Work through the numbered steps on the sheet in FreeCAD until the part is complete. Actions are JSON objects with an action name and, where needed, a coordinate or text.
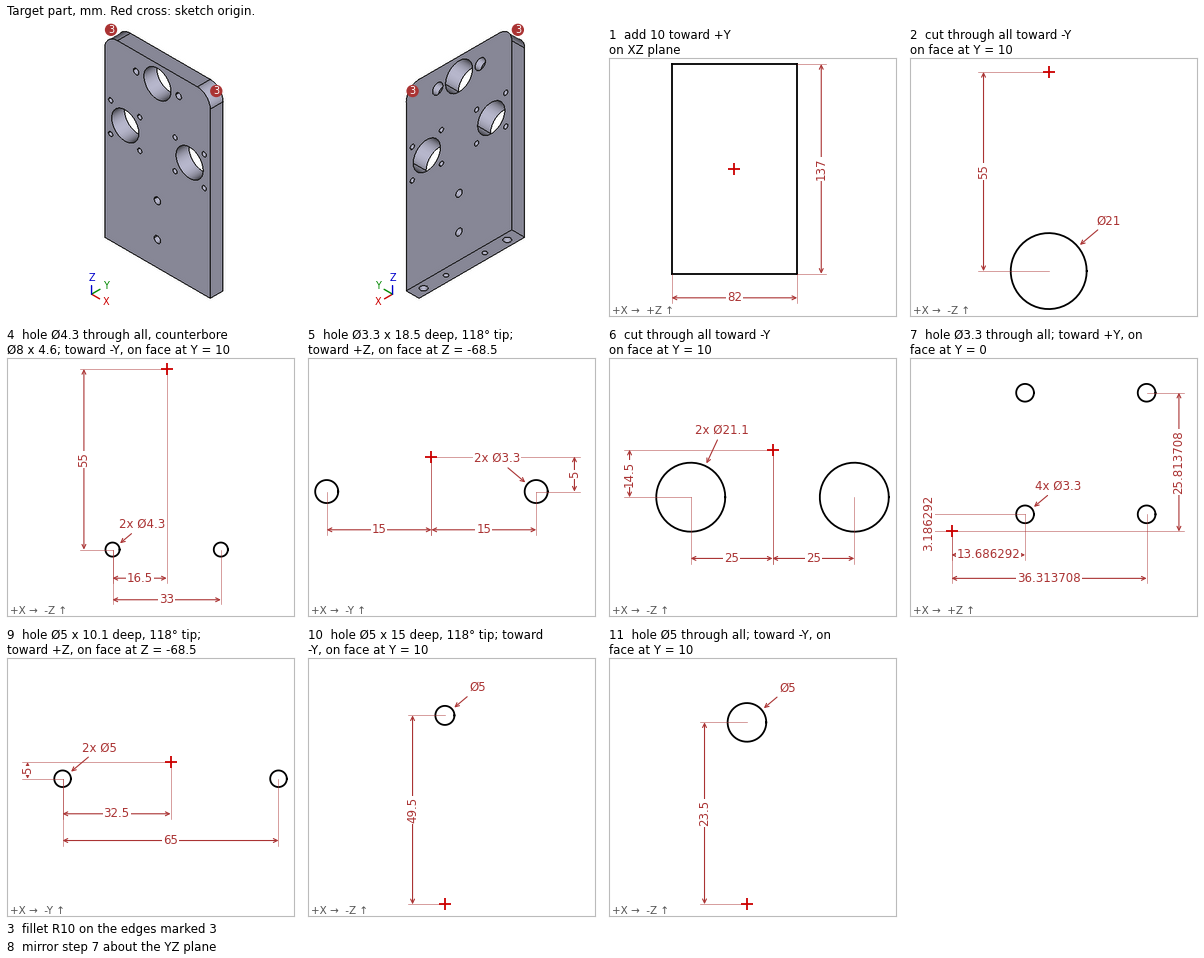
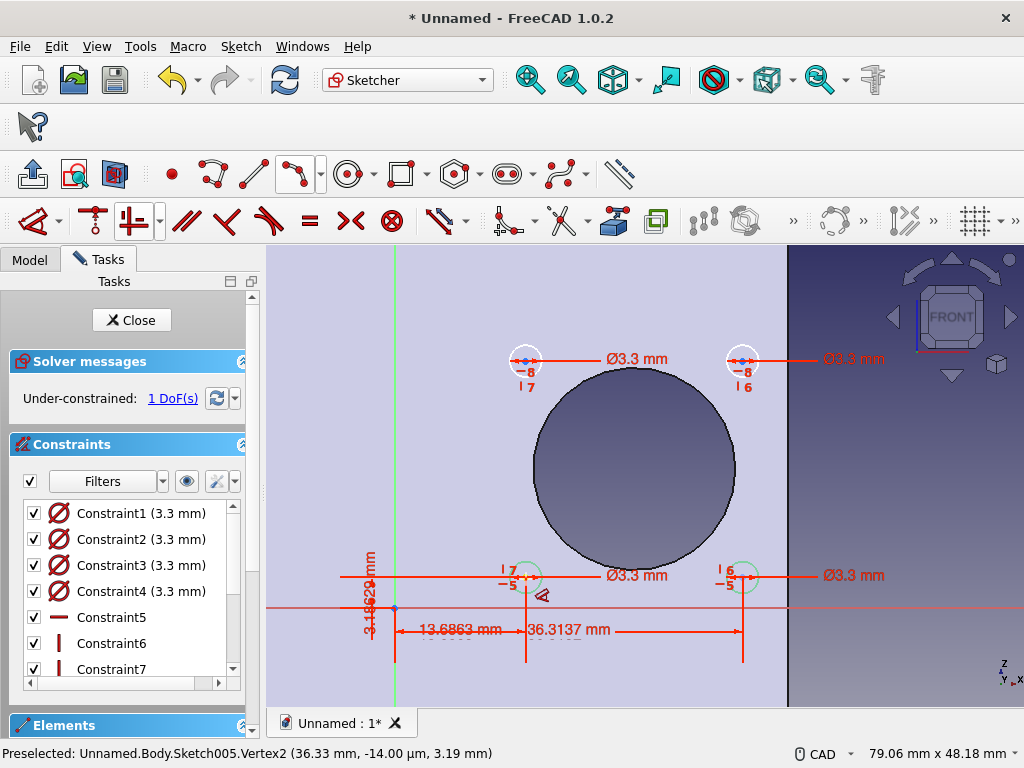
{"action": "left_click", "coordinate": [743, 361]}
{"action": "left_click", "coordinate": [361, 485]}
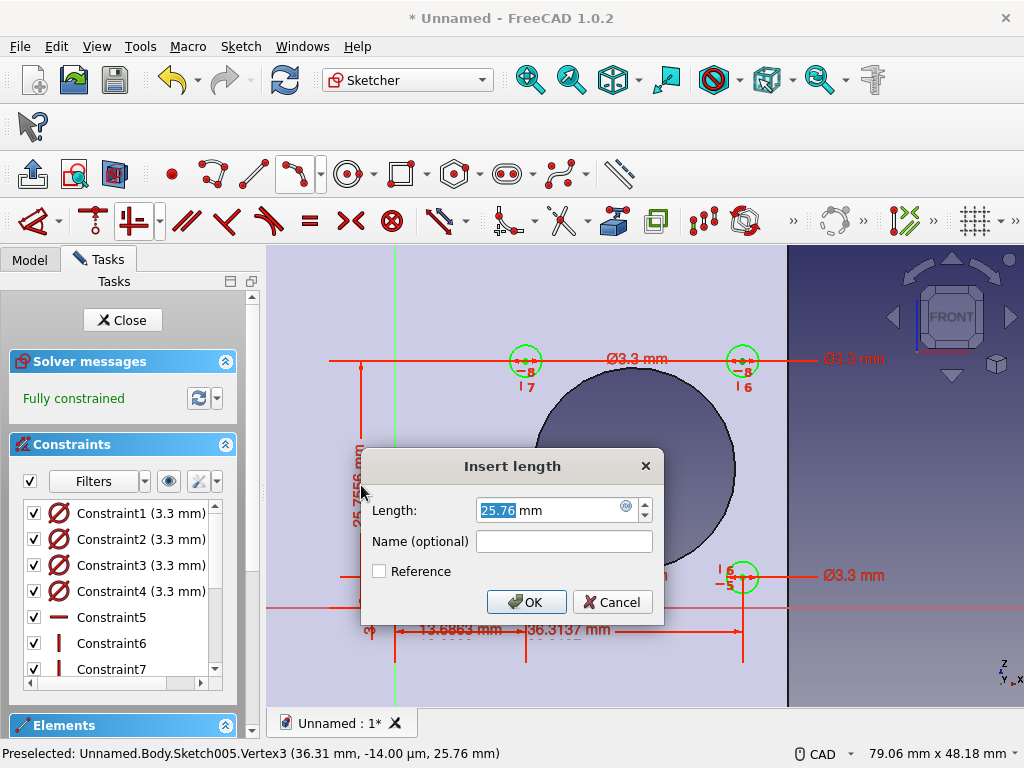
{"action": "type", "text": "25.813708"}
{"action": "key", "text": "Return"}
{"action": "key", "text": "Escape"}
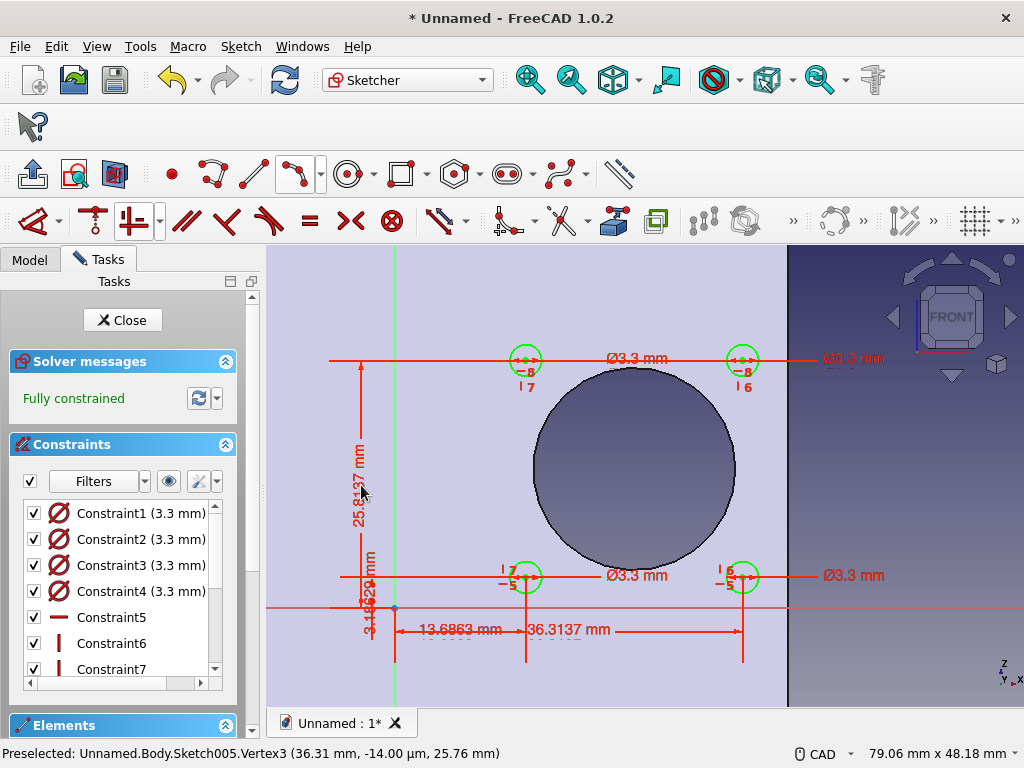
{"action": "left_click", "coordinate": [123, 320]}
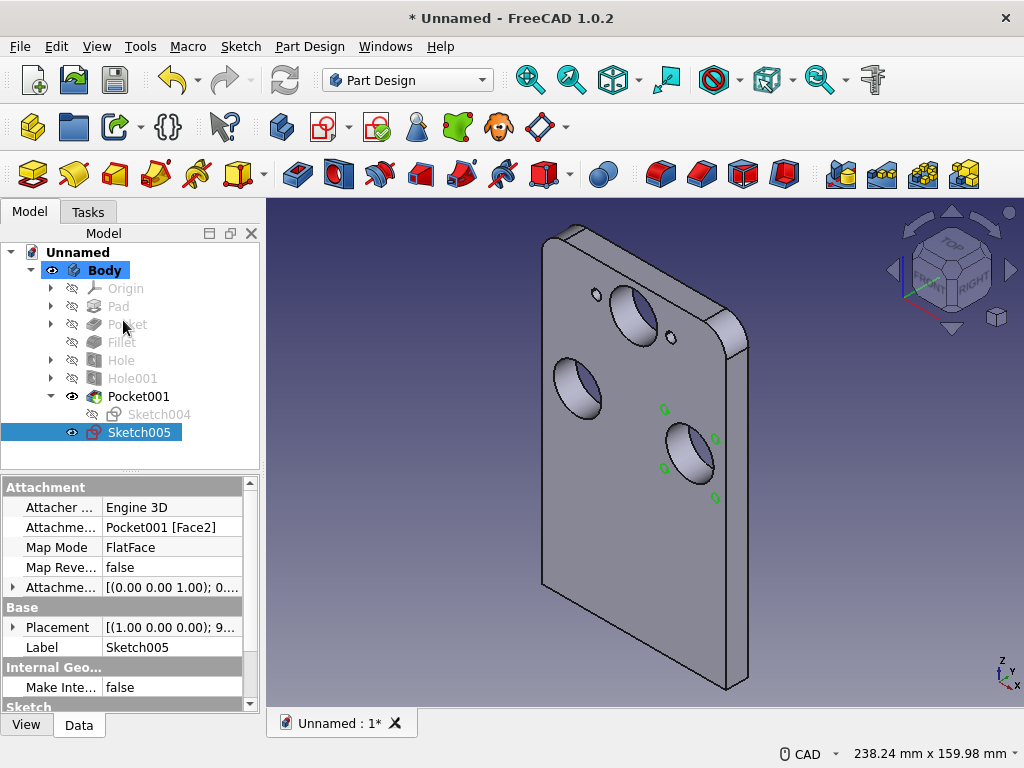
{"action": "left_click", "coordinate": [339, 174]}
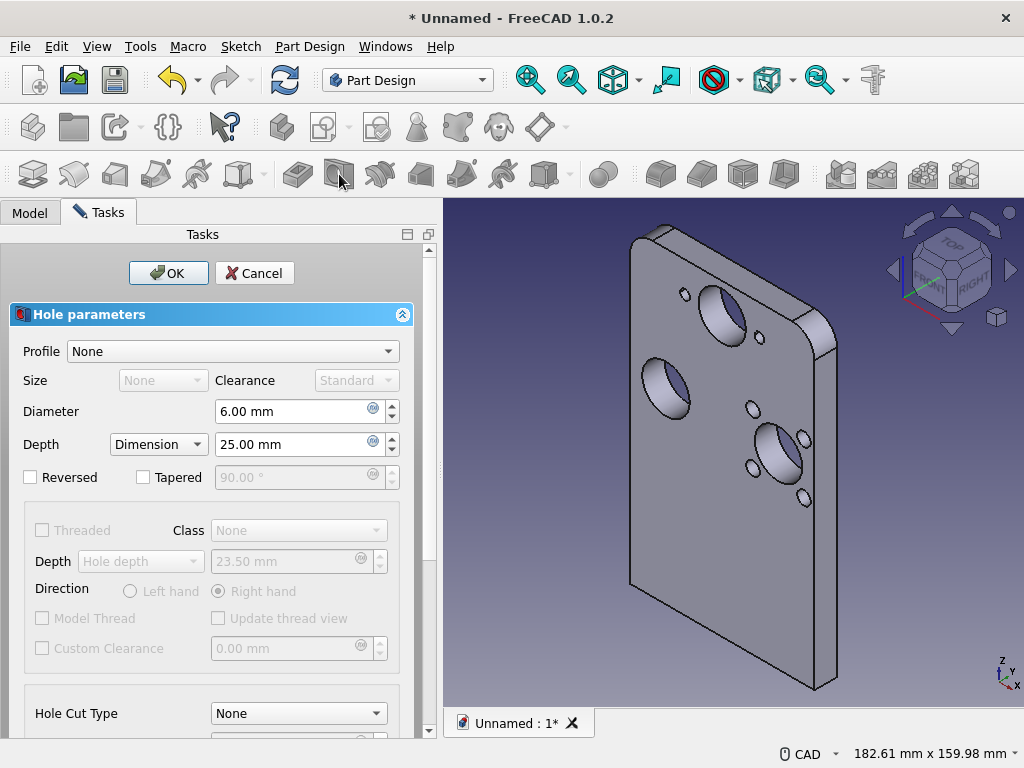
{"action": "triple_click", "coordinate": [300, 412]}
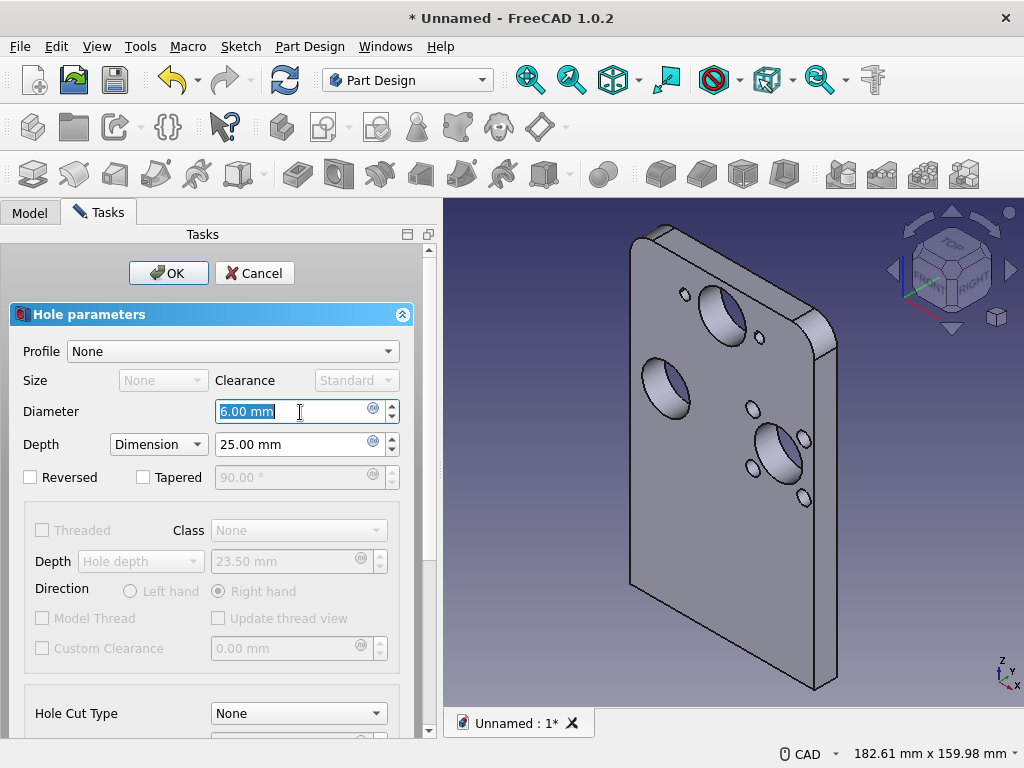
{"action": "type", "text": "3.3"}
{"action": "key", "text": "Tab"}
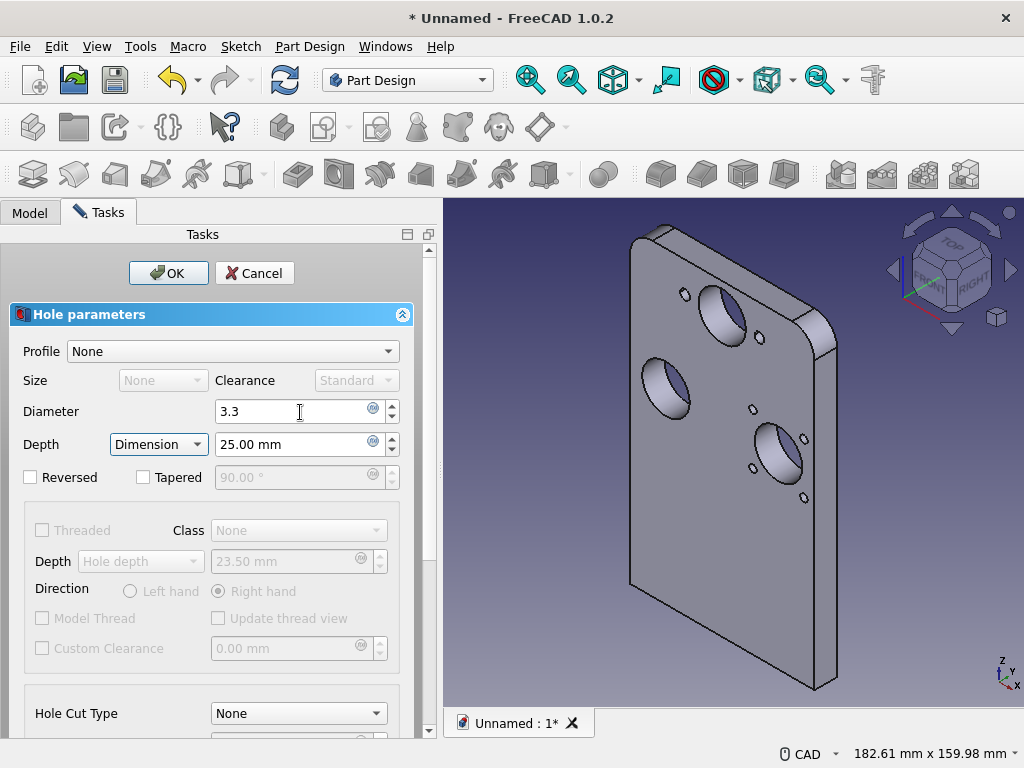
{"action": "left_click", "coordinate": [160, 444]}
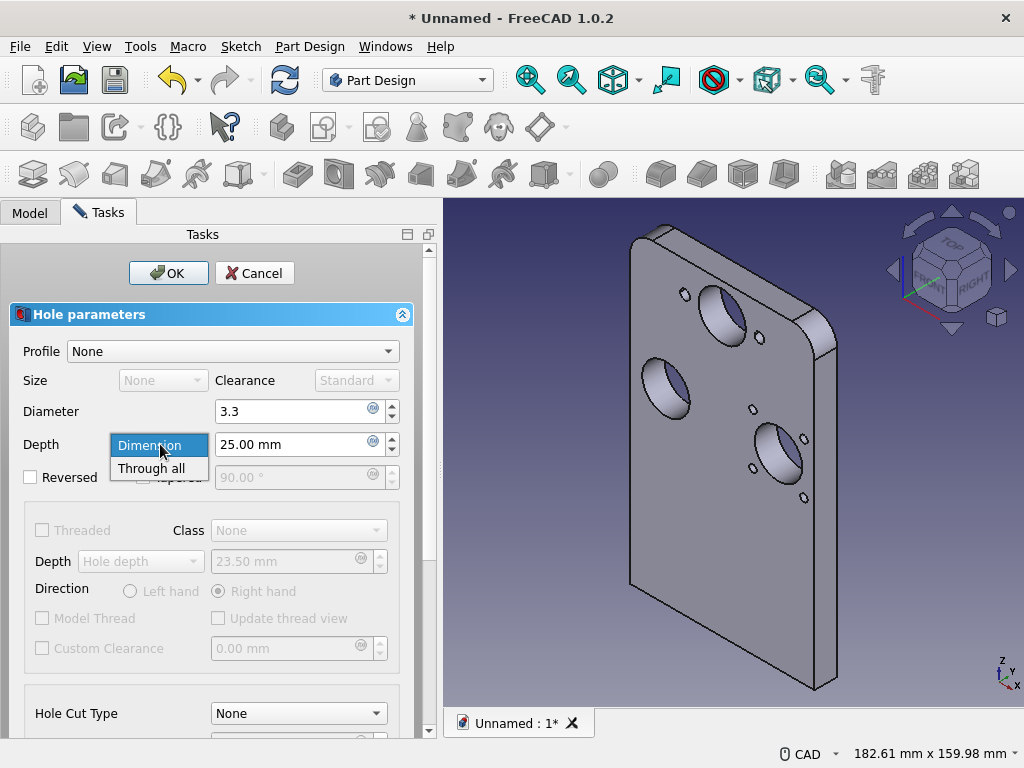
{"action": "left_click", "coordinate": [158, 468]}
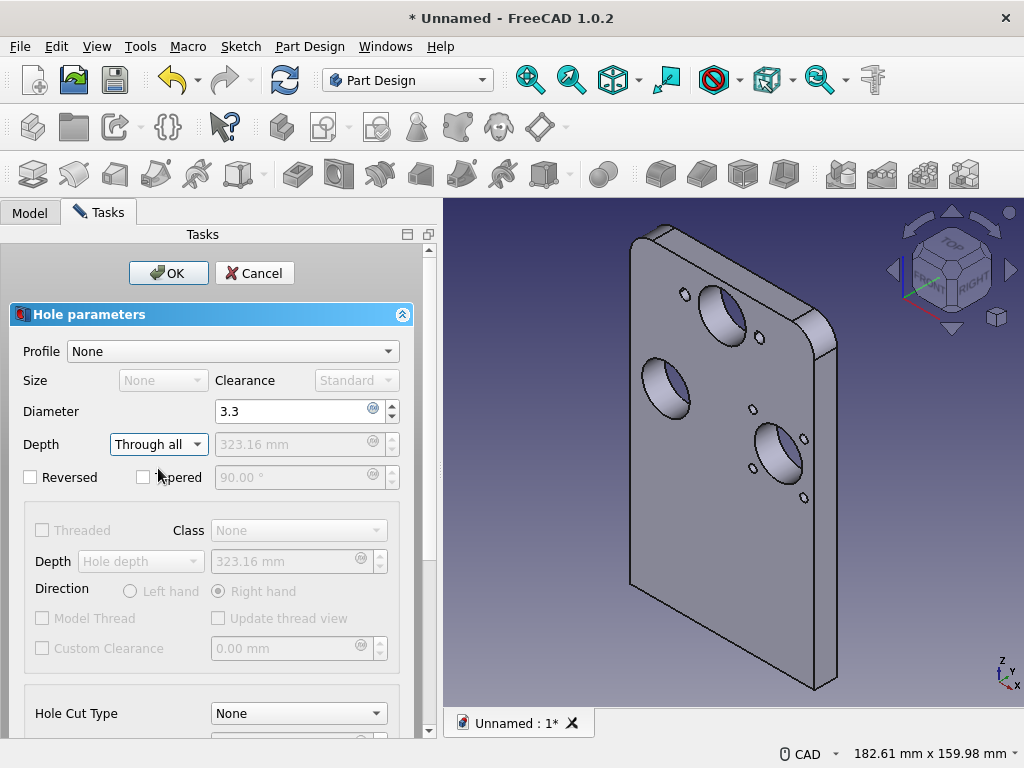
{"action": "left_click", "coordinate": [169, 273]}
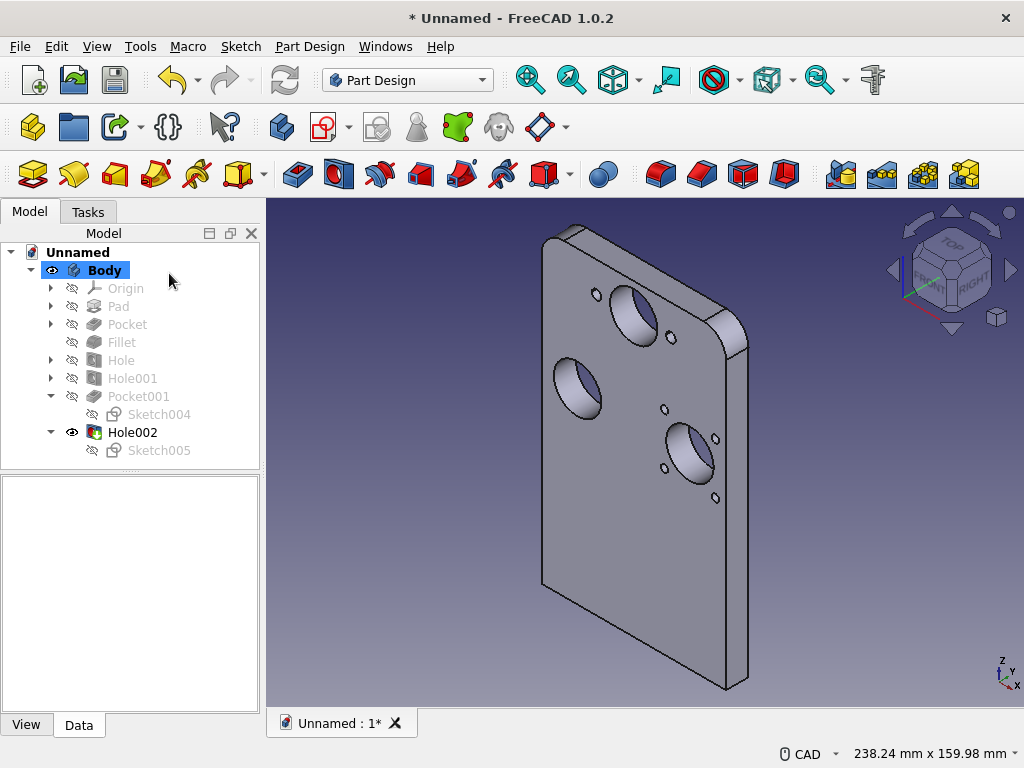
{"action": "left_click", "coordinate": [117, 432]}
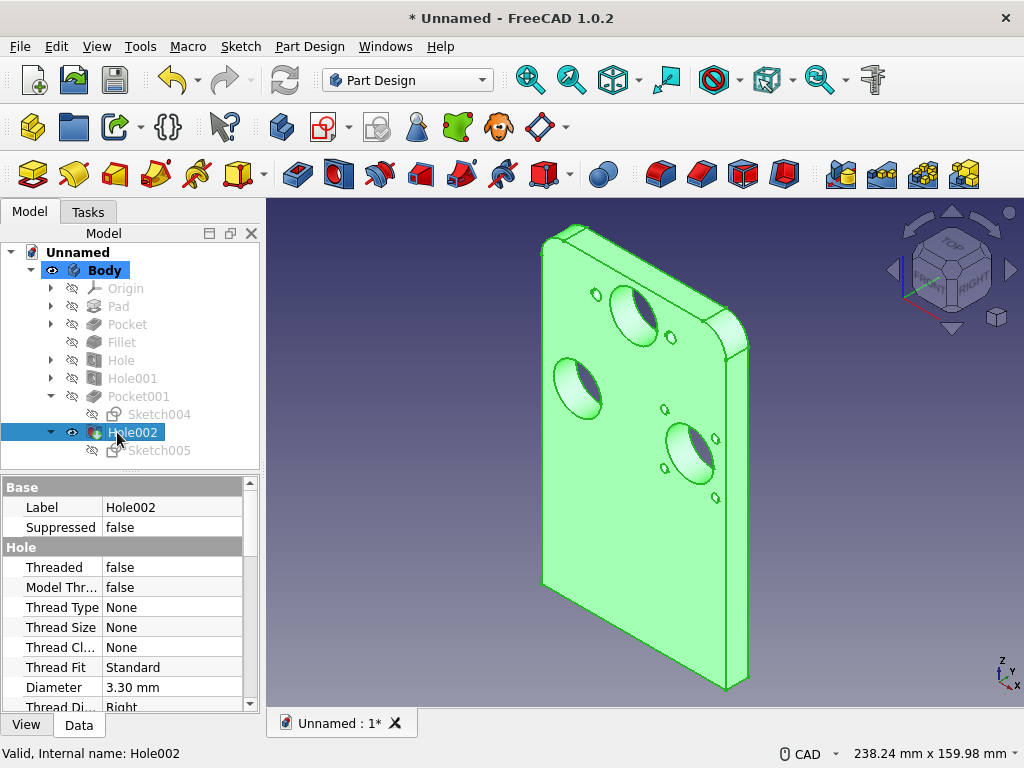
{"action": "left_click", "coordinate": [841, 174]}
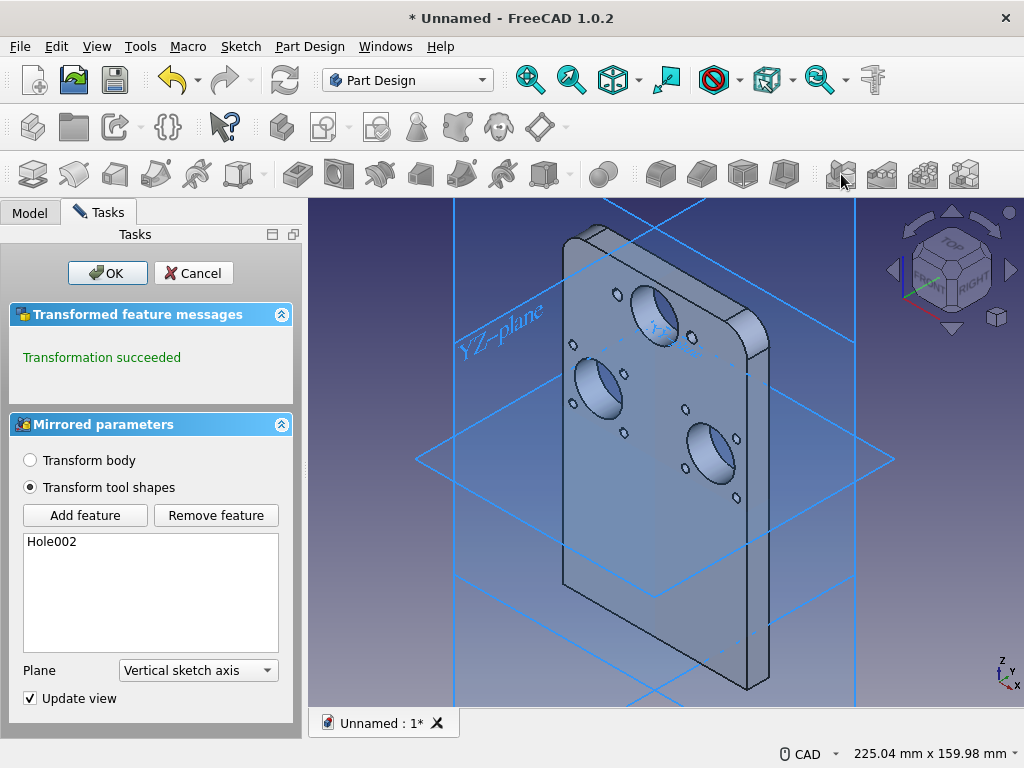
{"action": "left_click", "coordinate": [199, 670]}